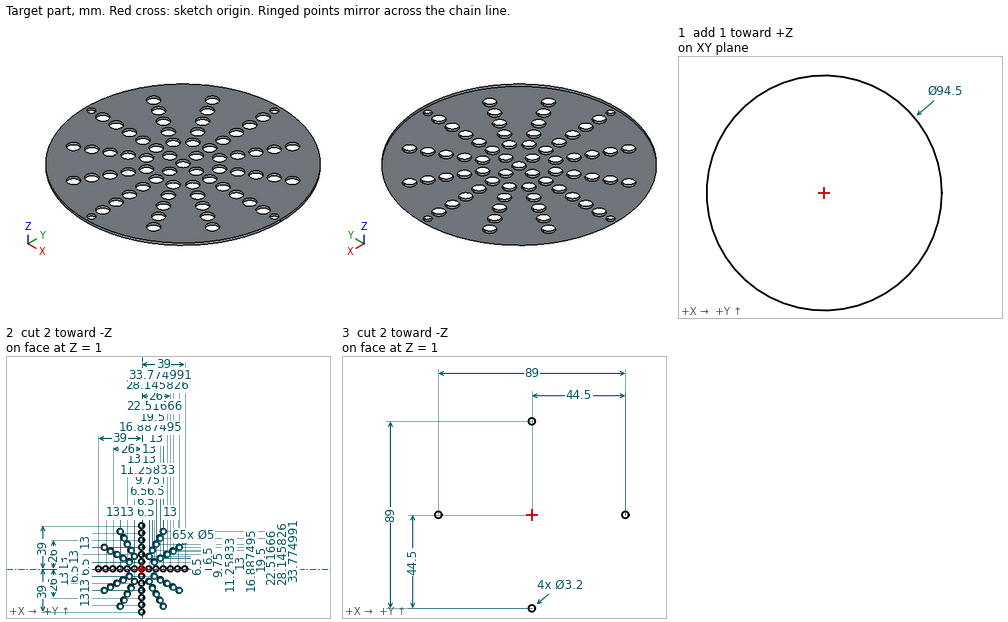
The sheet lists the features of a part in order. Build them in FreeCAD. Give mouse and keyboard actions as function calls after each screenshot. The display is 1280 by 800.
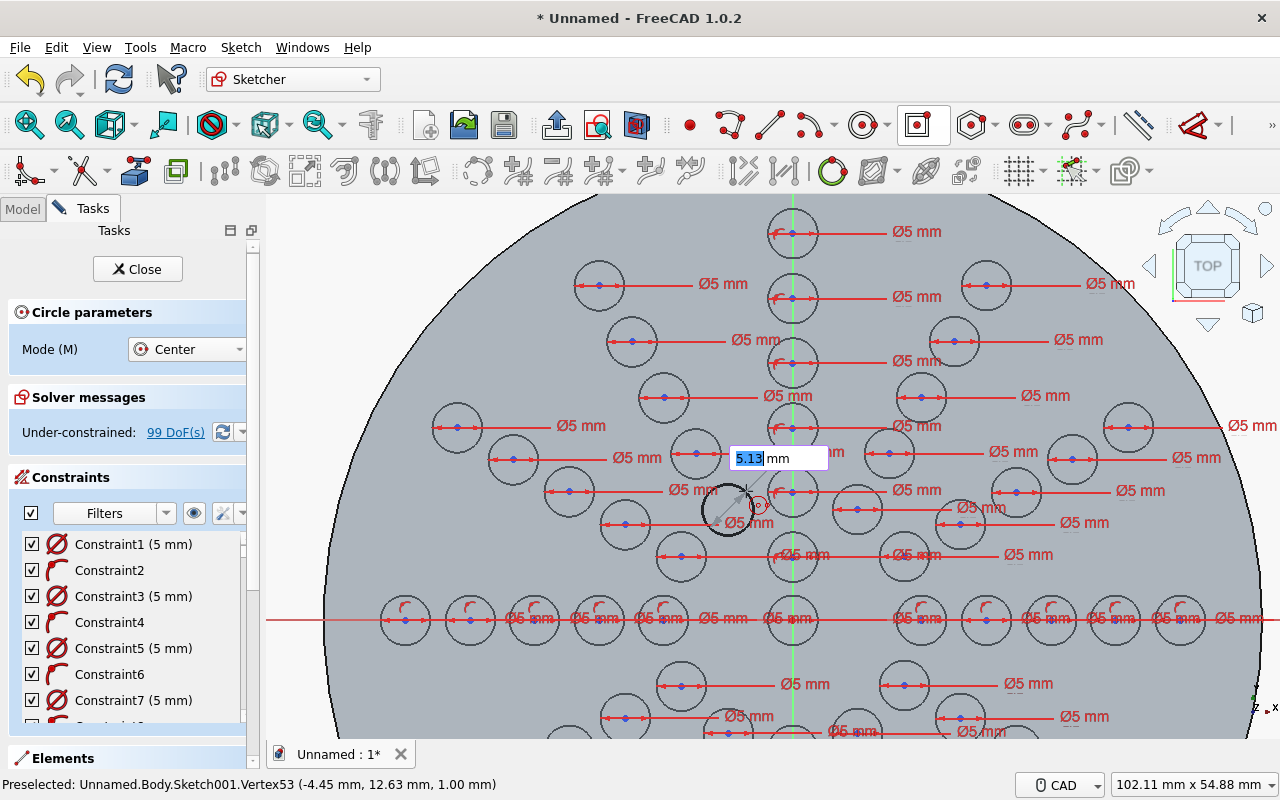
text(5)
key(Return)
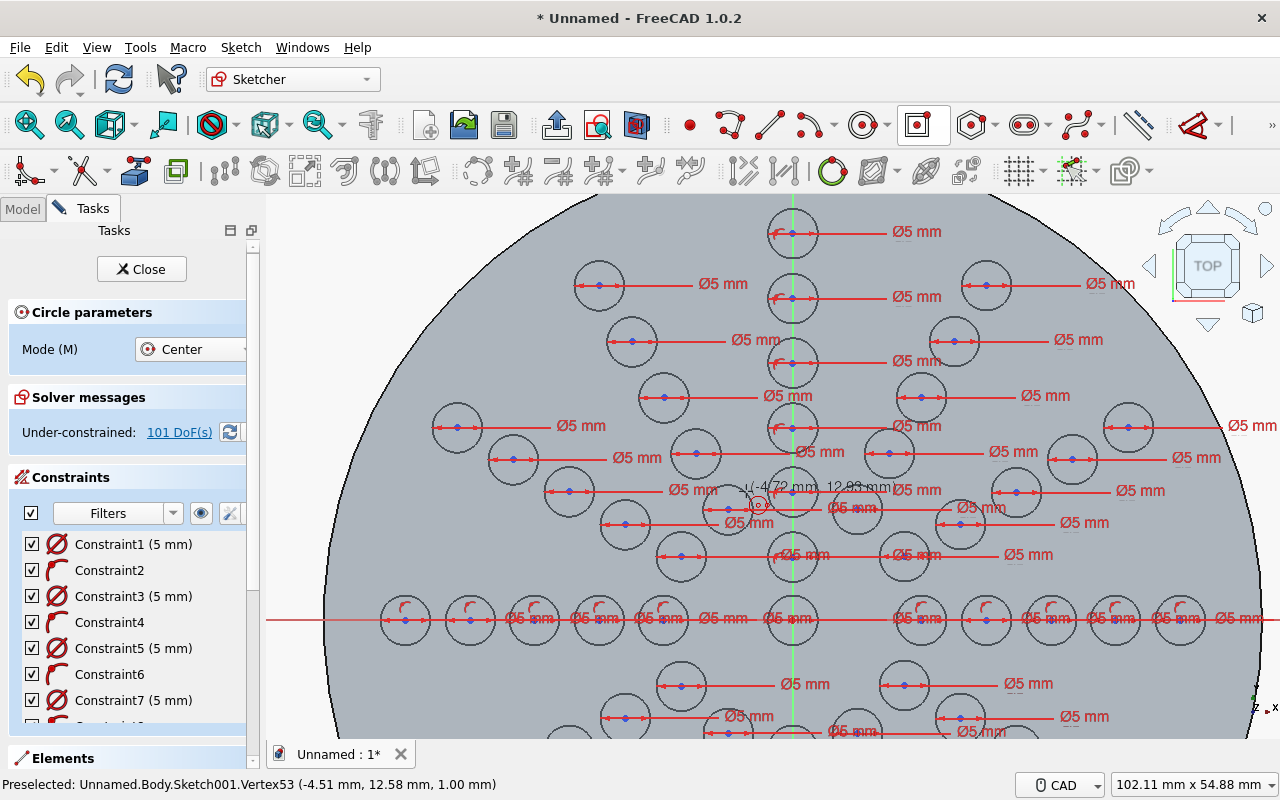
click(857, 620)
move(875, 603)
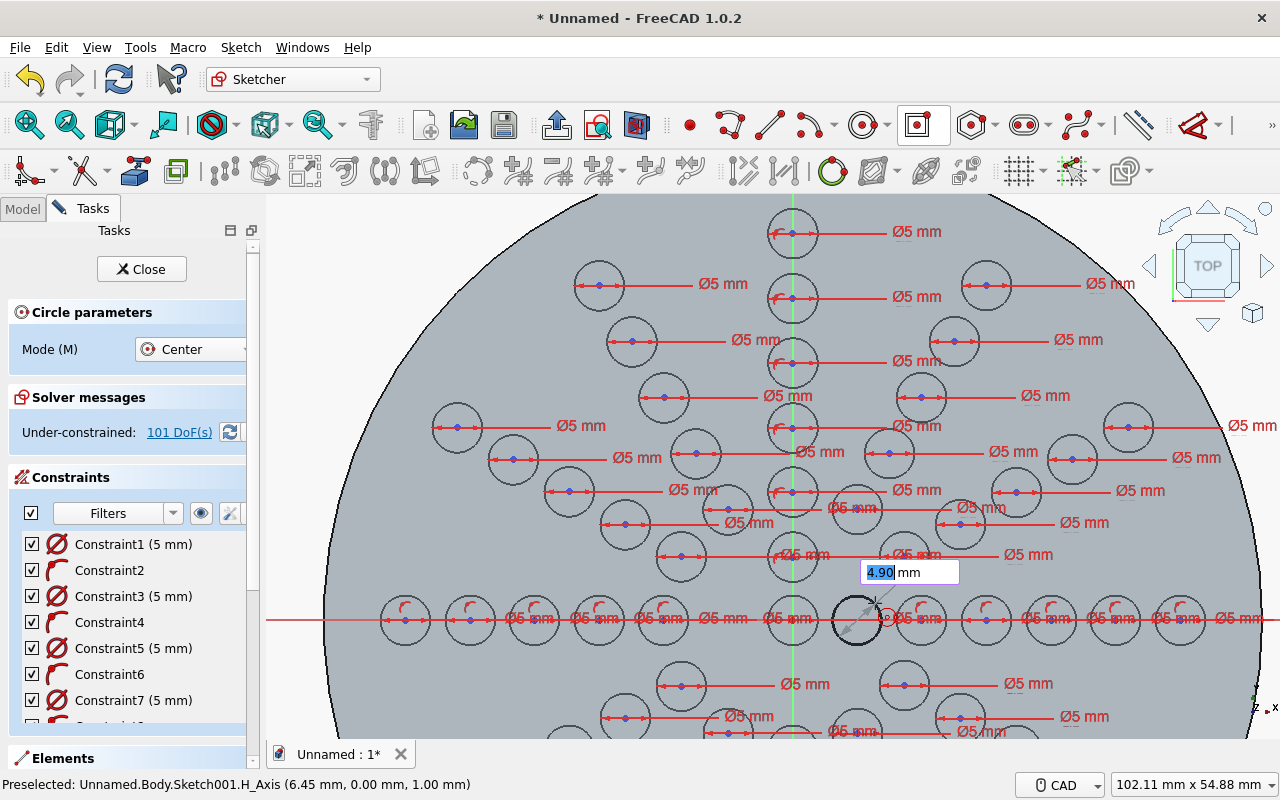
text(5)
key(Return)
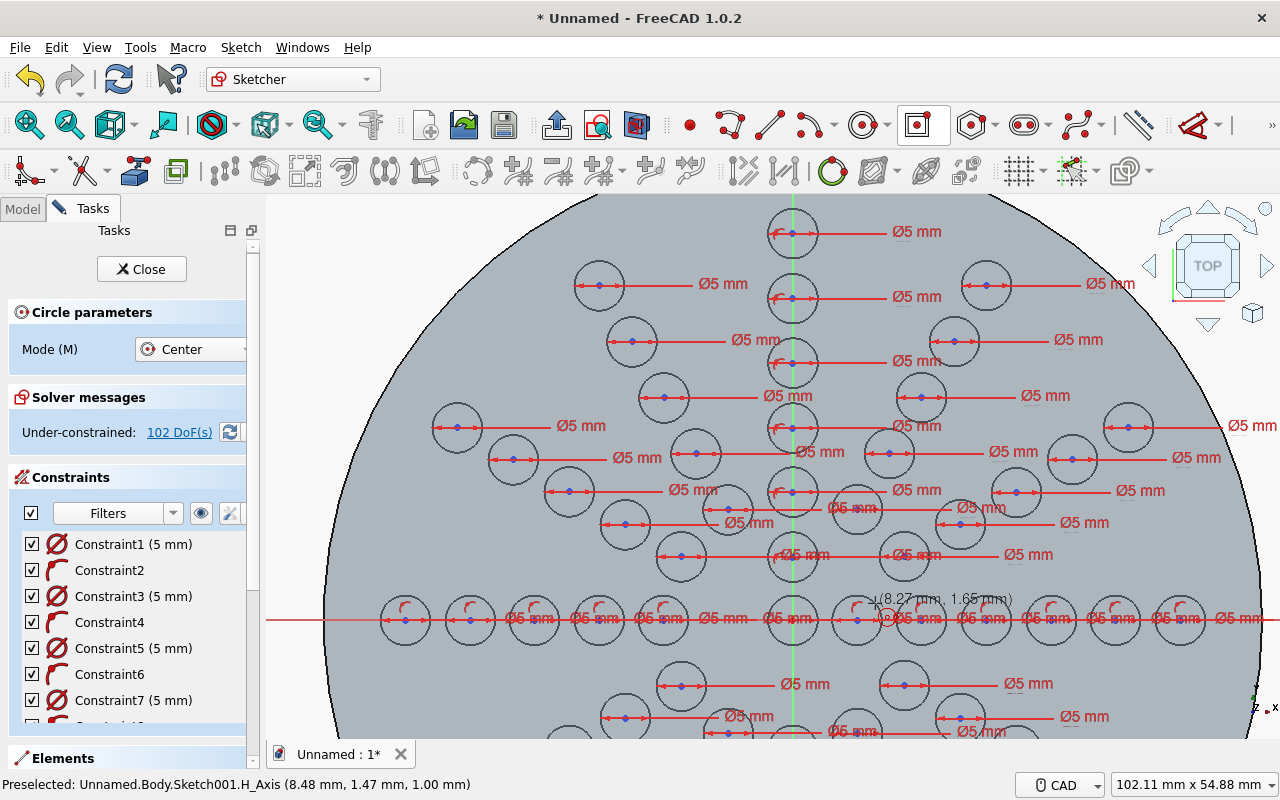
click(793, 685)
move(810, 667)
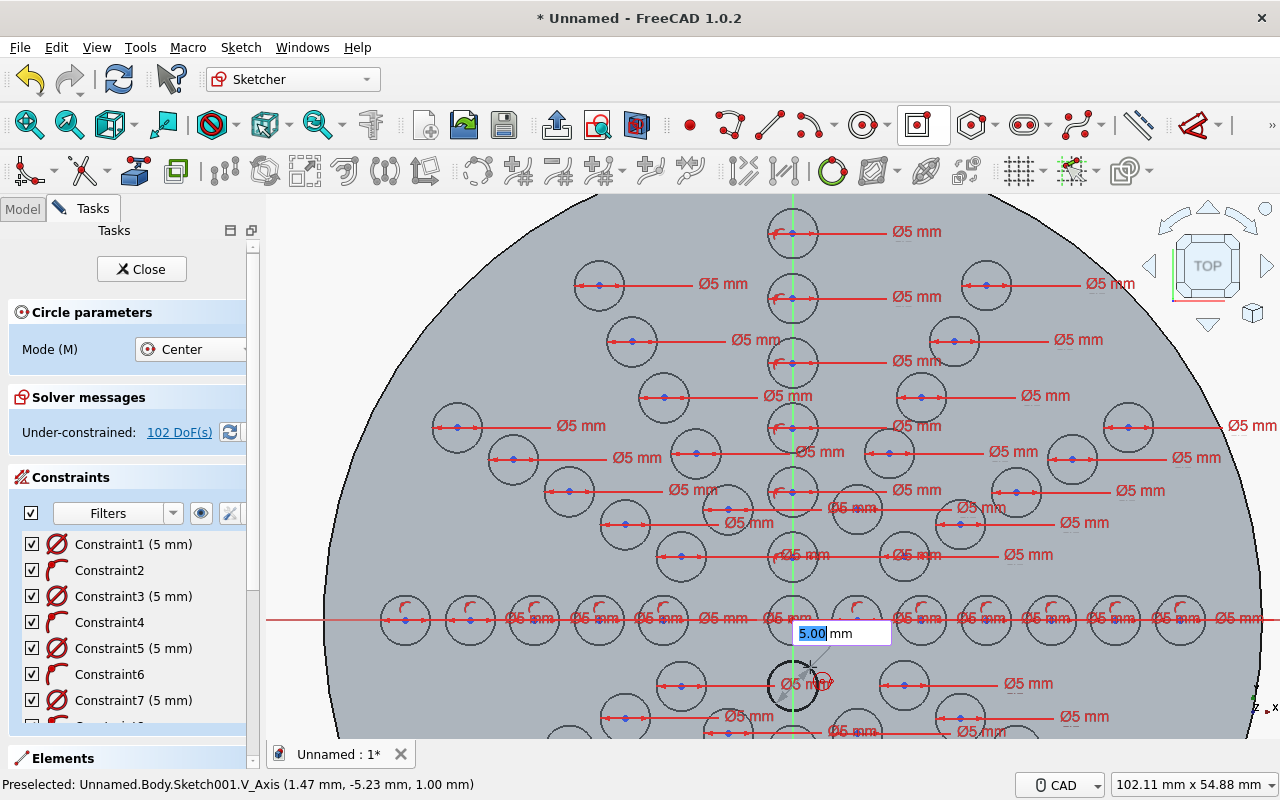
text(5)
key(Return)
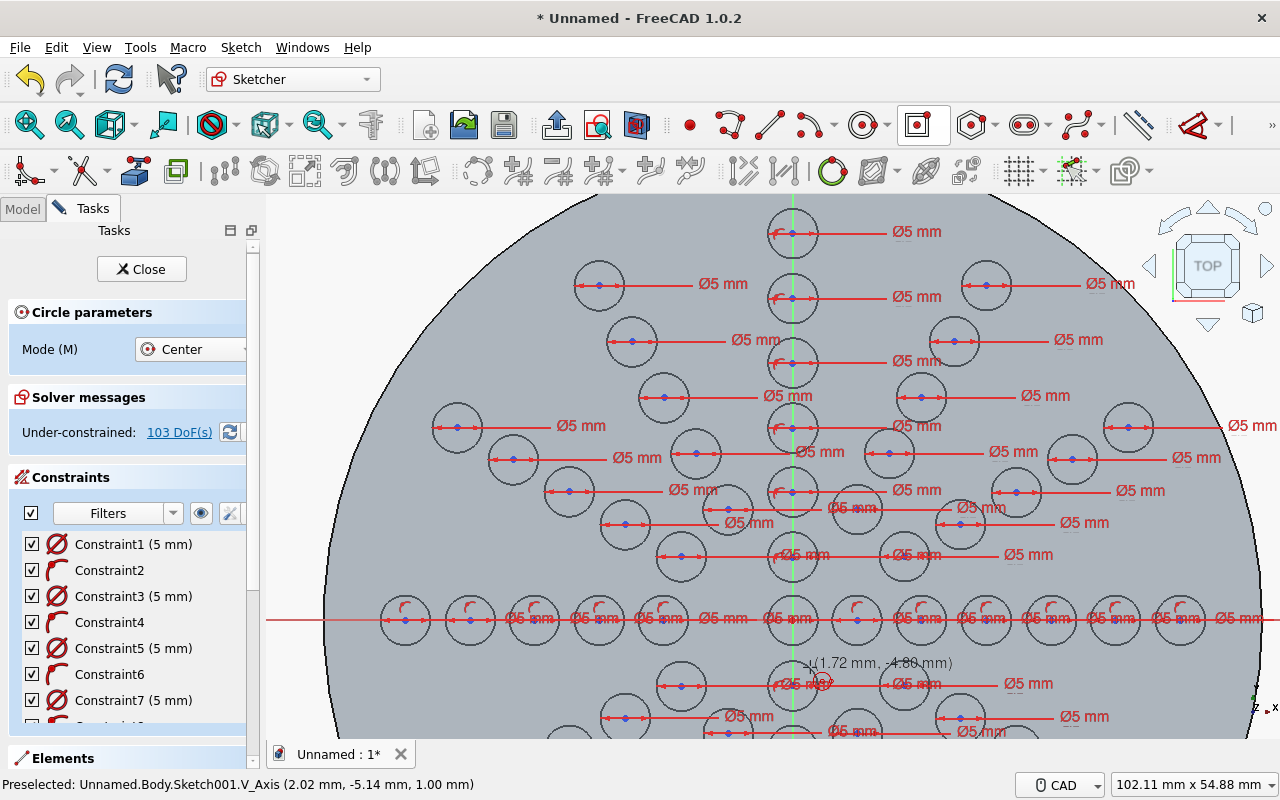
click(728, 620)
move(746, 603)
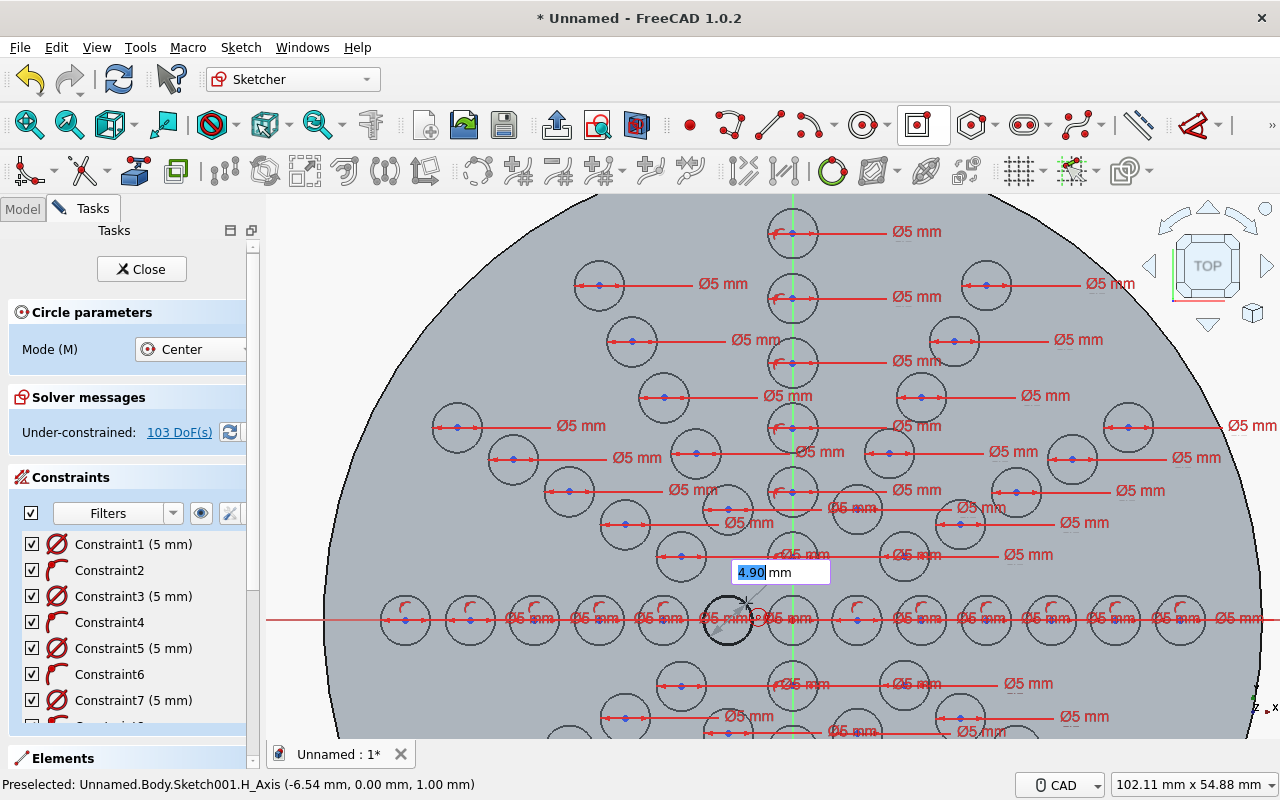
text(5)
key(Return)
key(Escape)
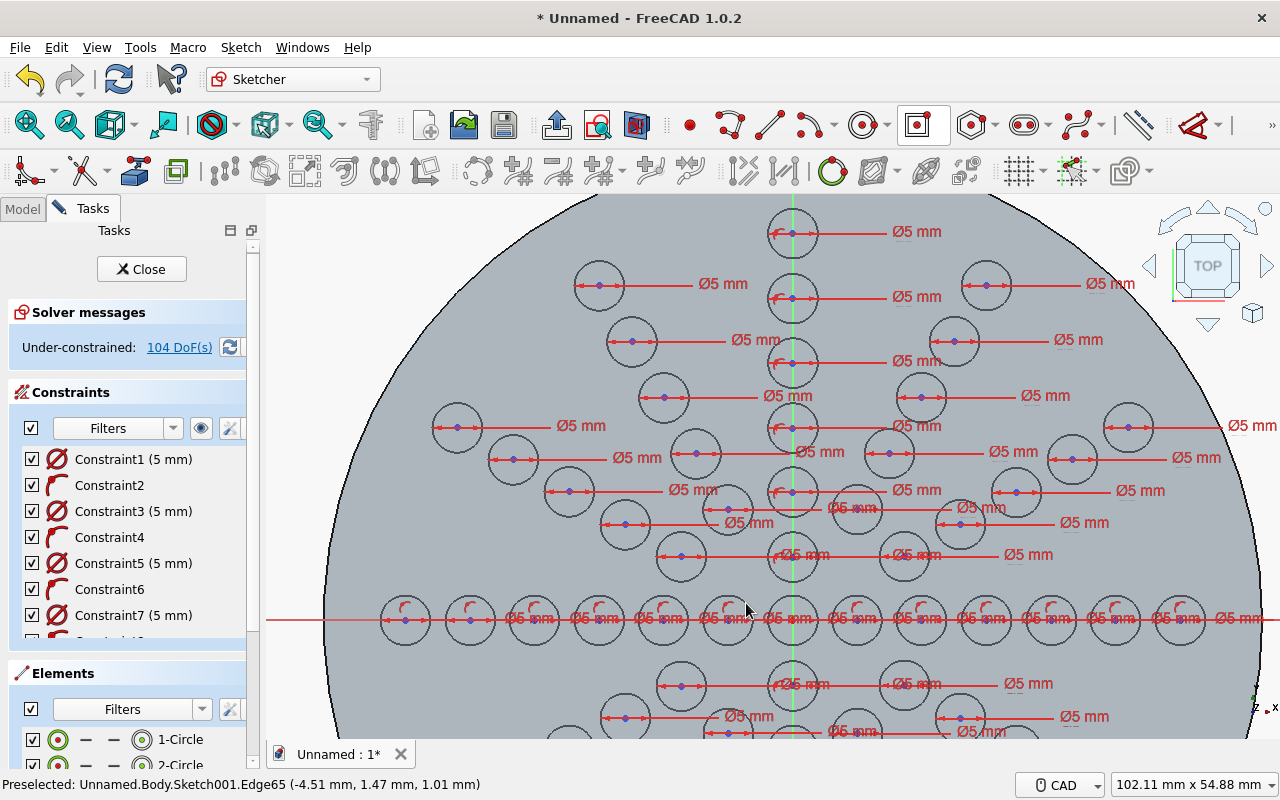
scroll(632, 341, down, 4)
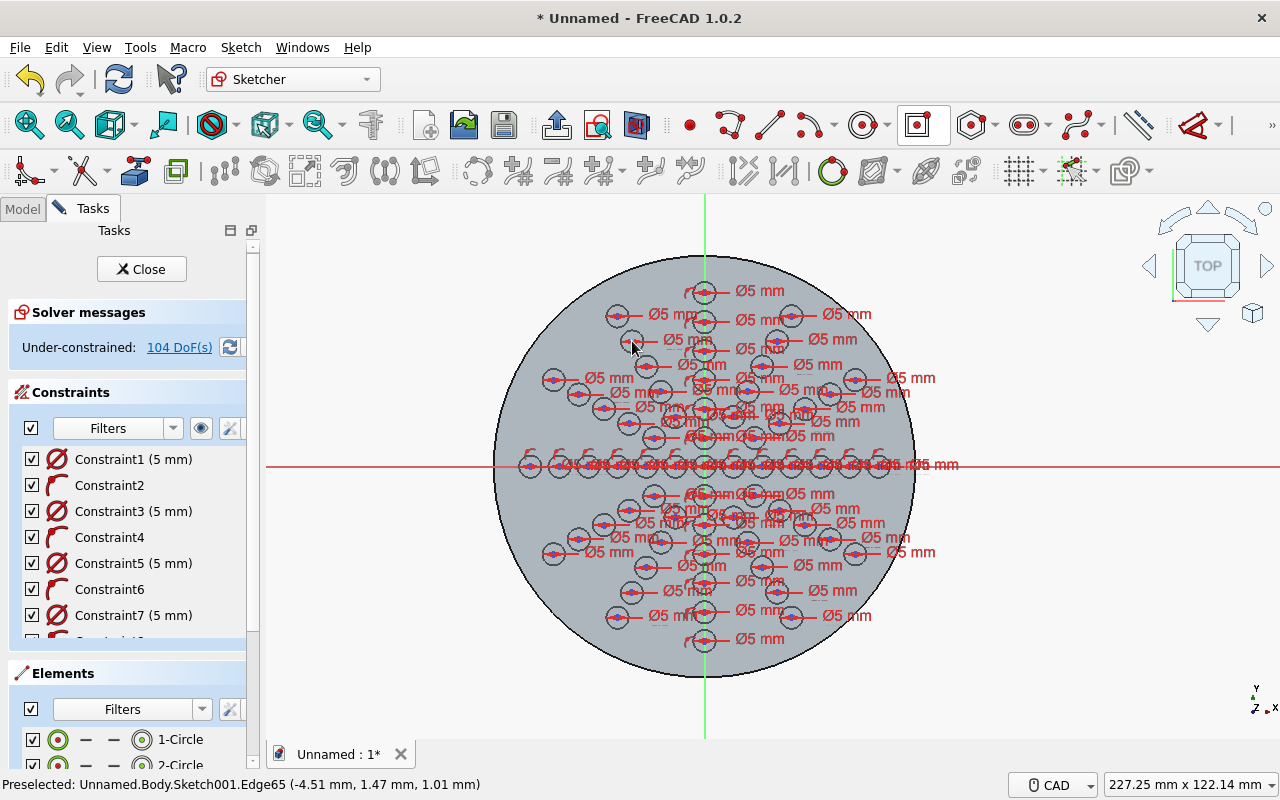
click(855, 380)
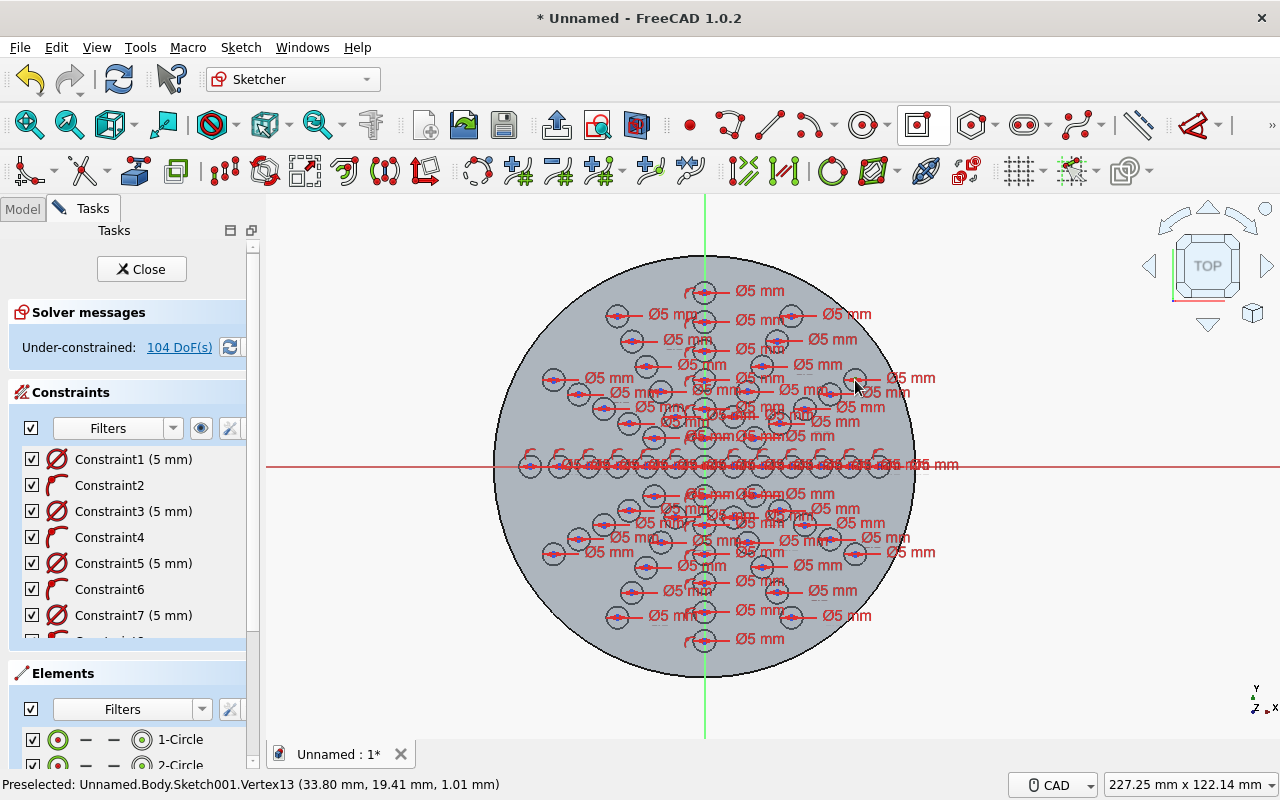
click(855, 554)